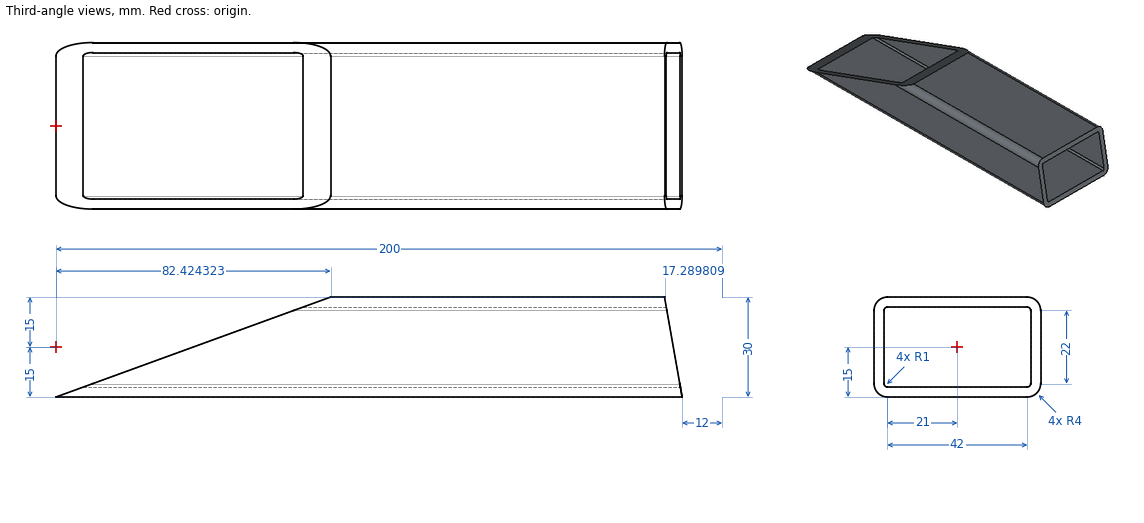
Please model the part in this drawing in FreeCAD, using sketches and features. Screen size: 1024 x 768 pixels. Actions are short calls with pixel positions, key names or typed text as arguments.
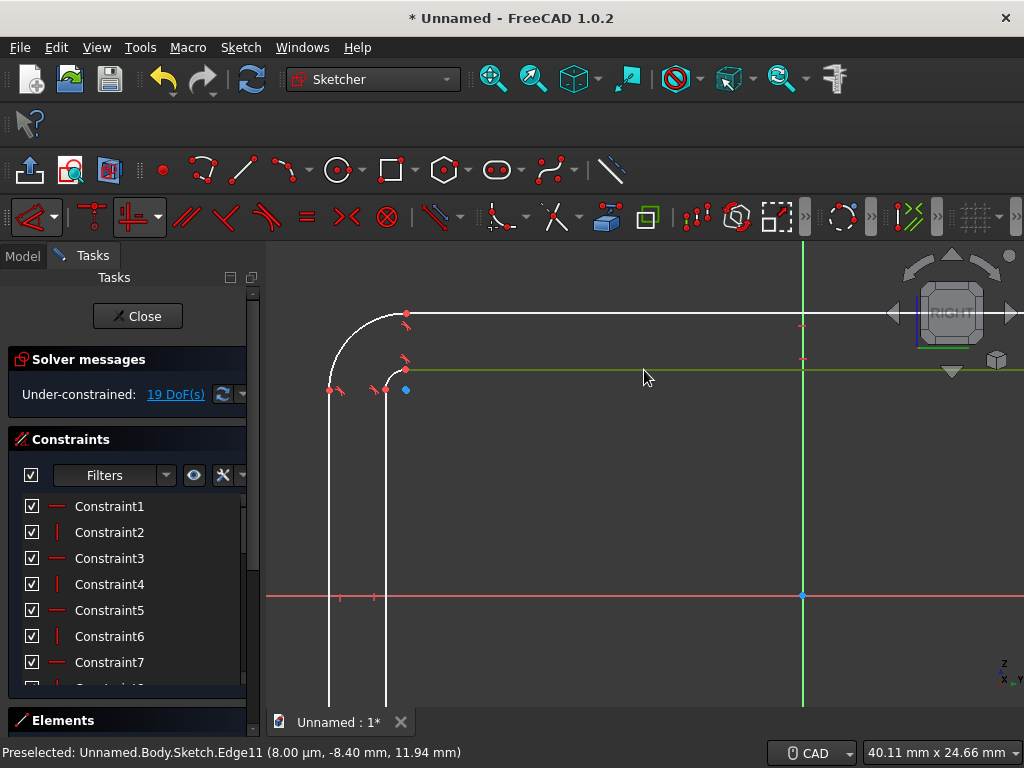
scroll(392, 375, down, 4)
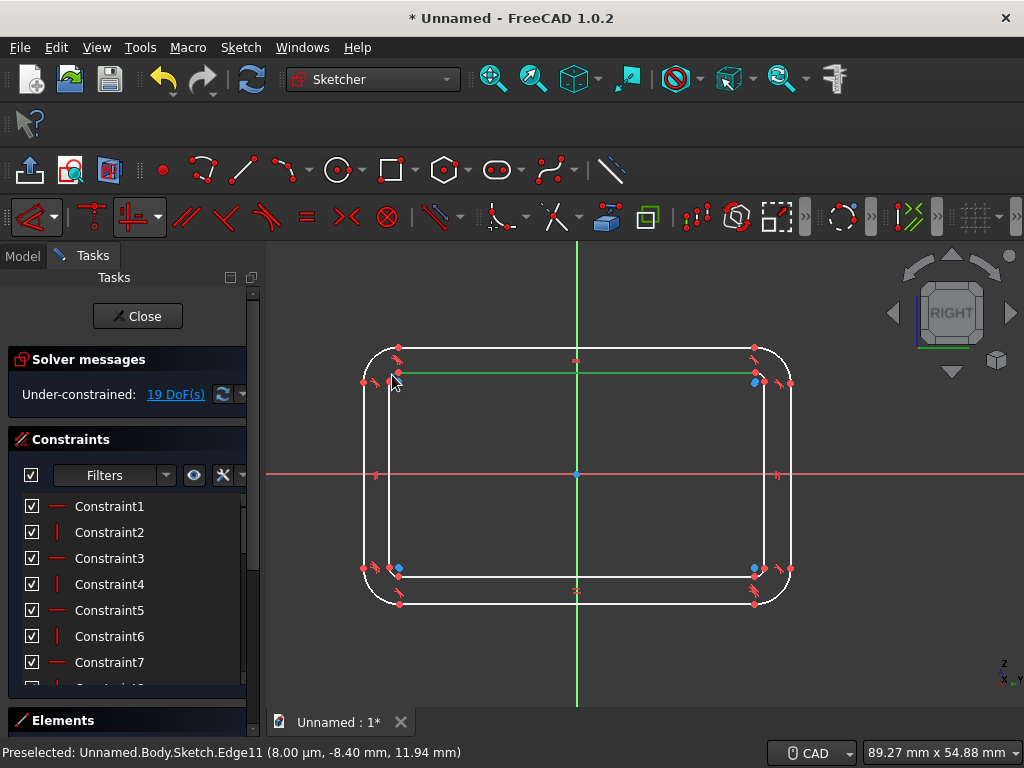
scroll(764, 377, up, 7)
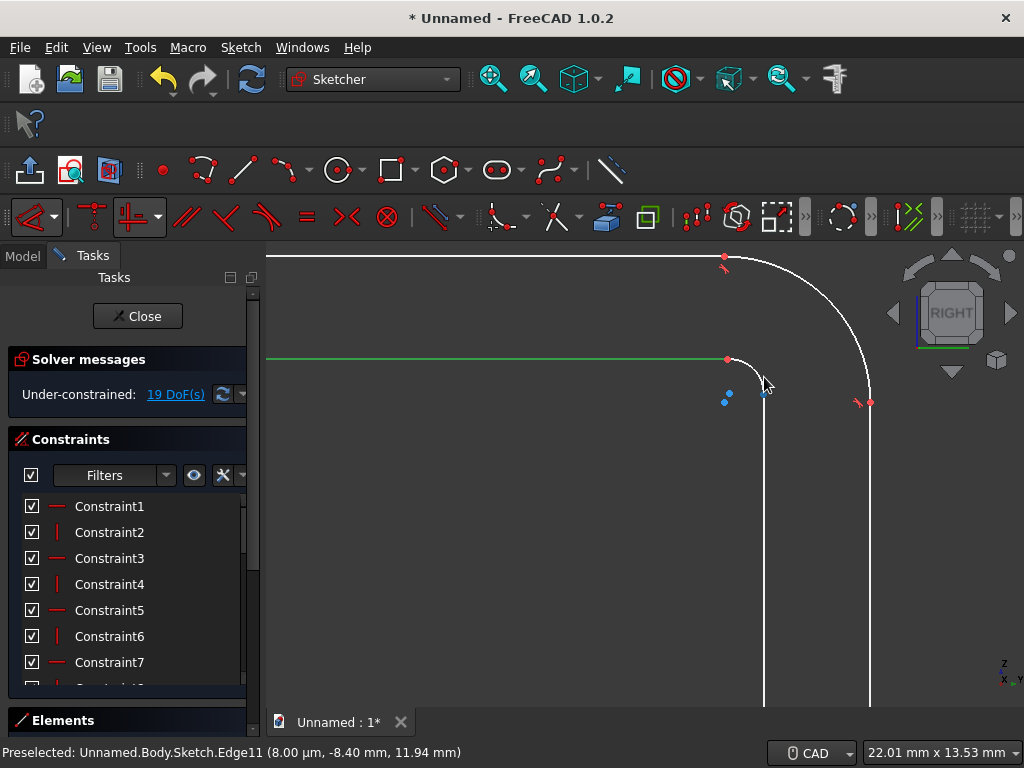
click(760, 378)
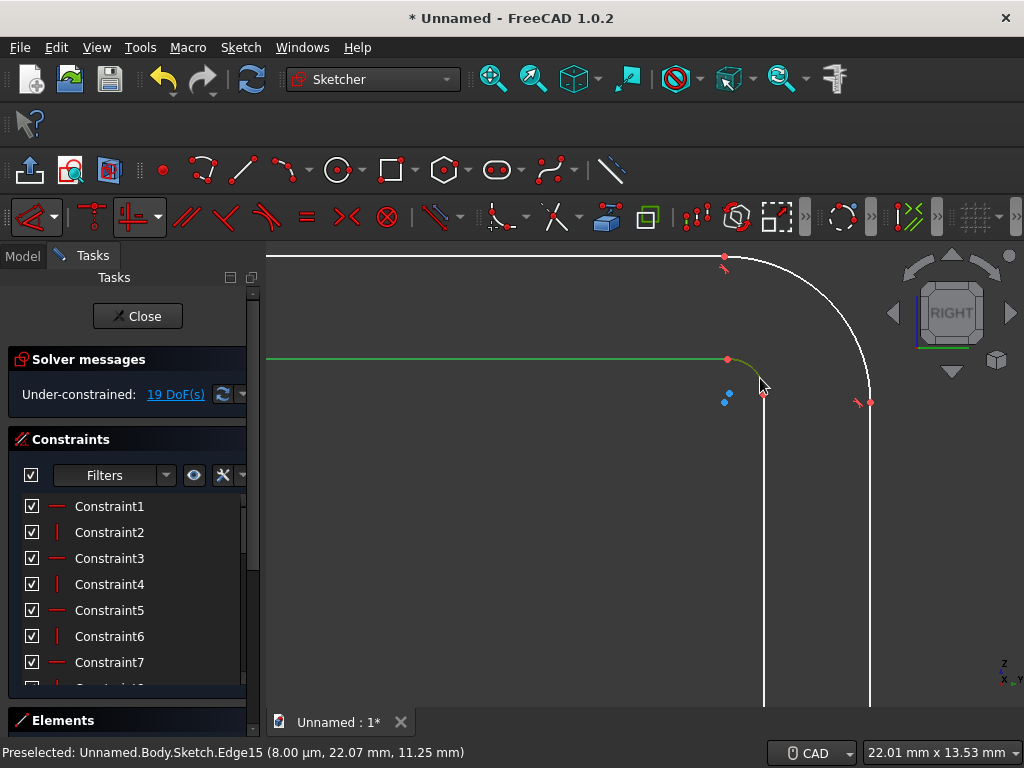
click(268, 218)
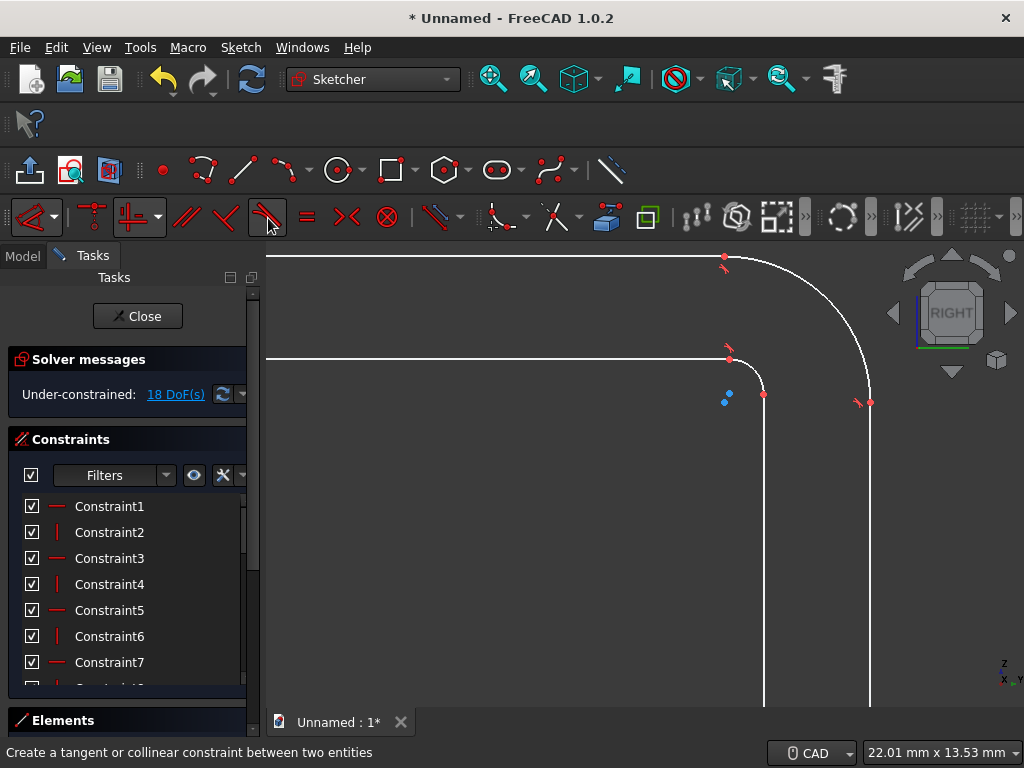
scroll(764, 377, down, 7)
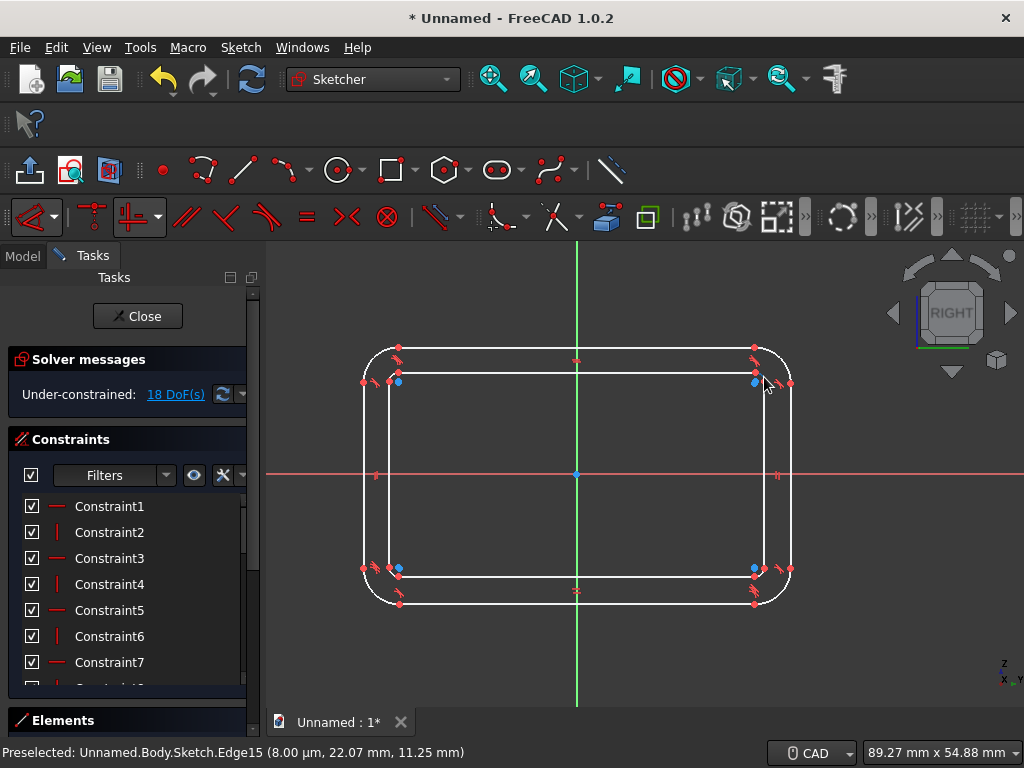
click(764, 437)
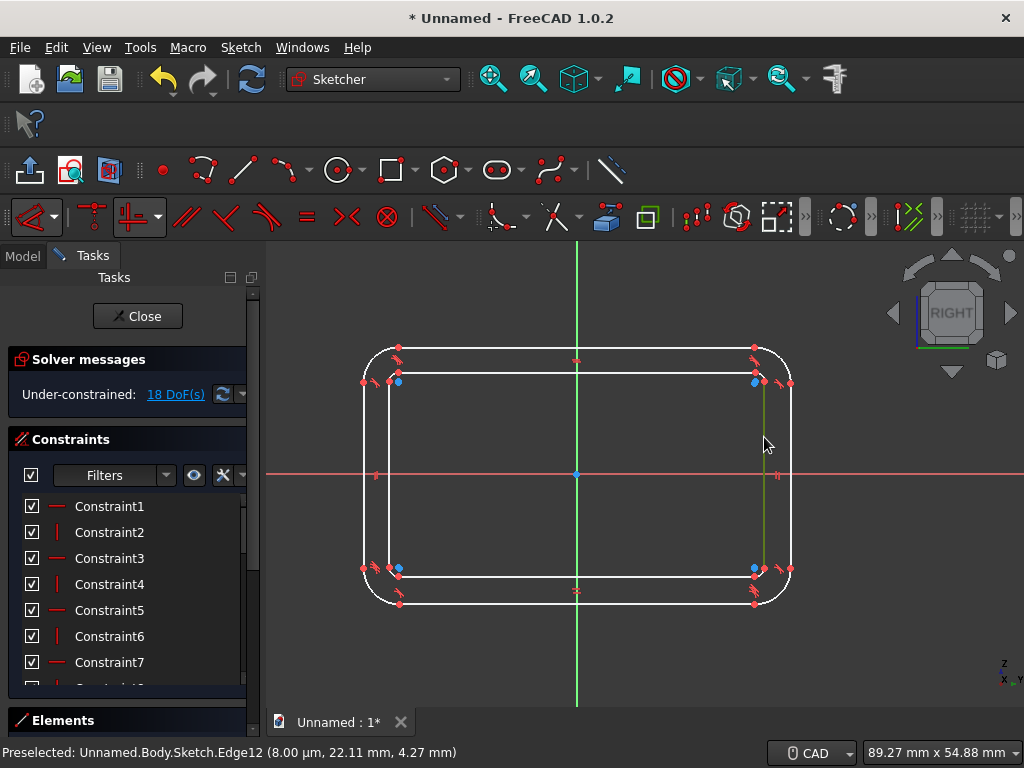
scroll(762, 375, up, 4)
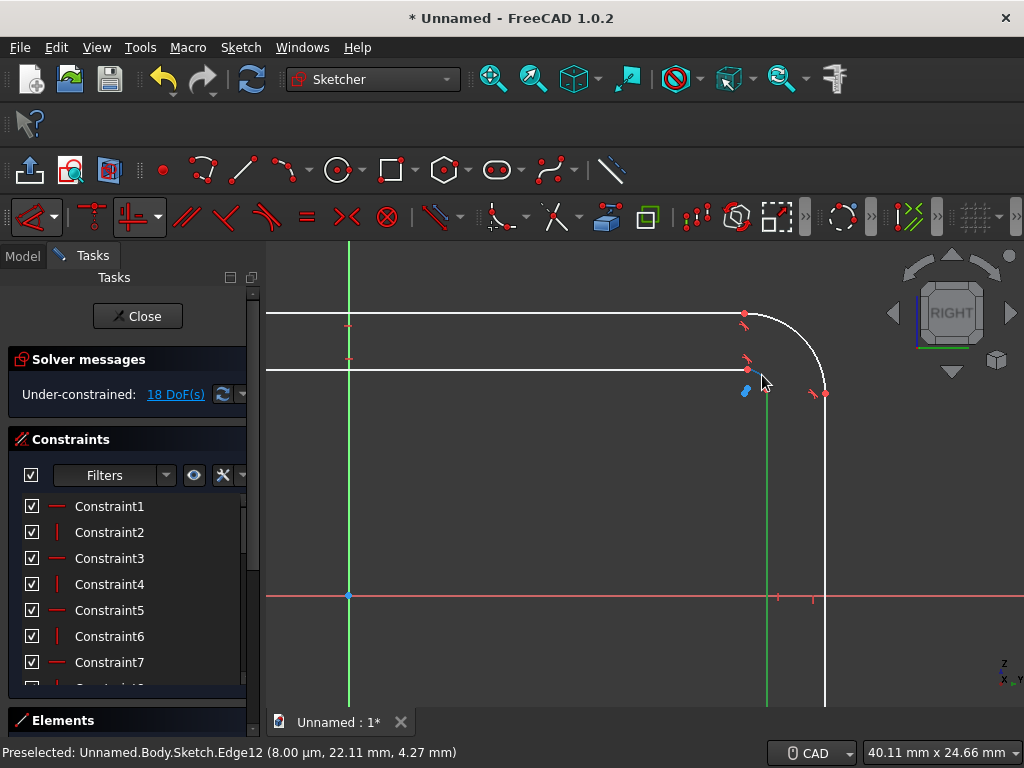
click(761, 376)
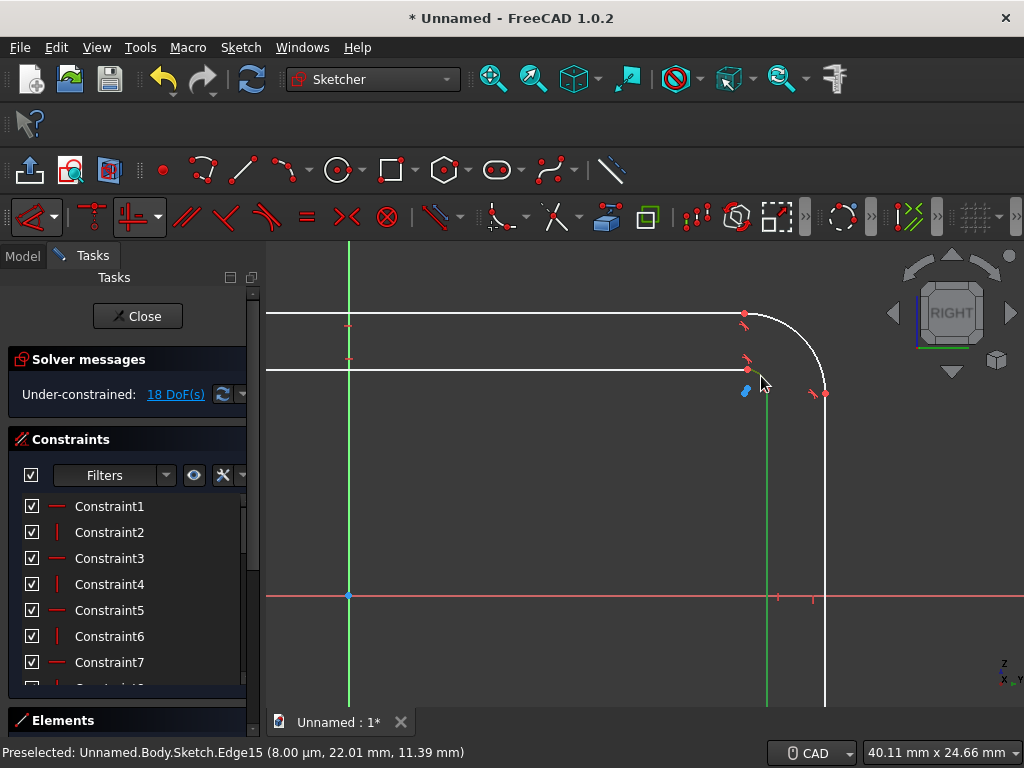
click(268, 218)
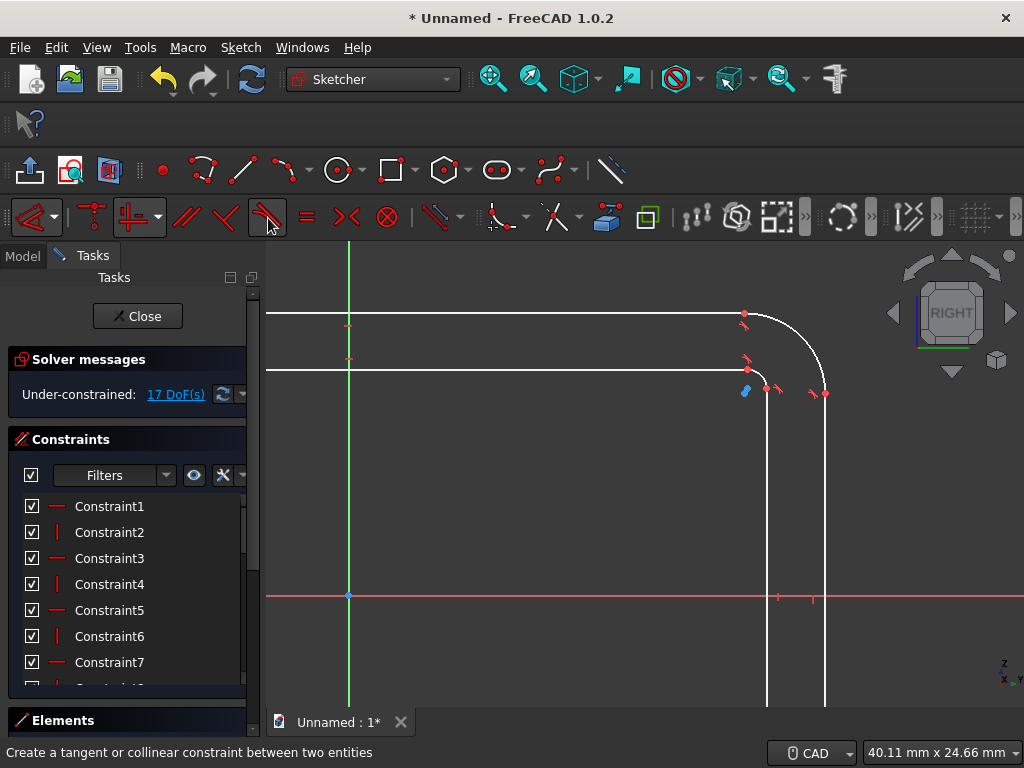
click(767, 513)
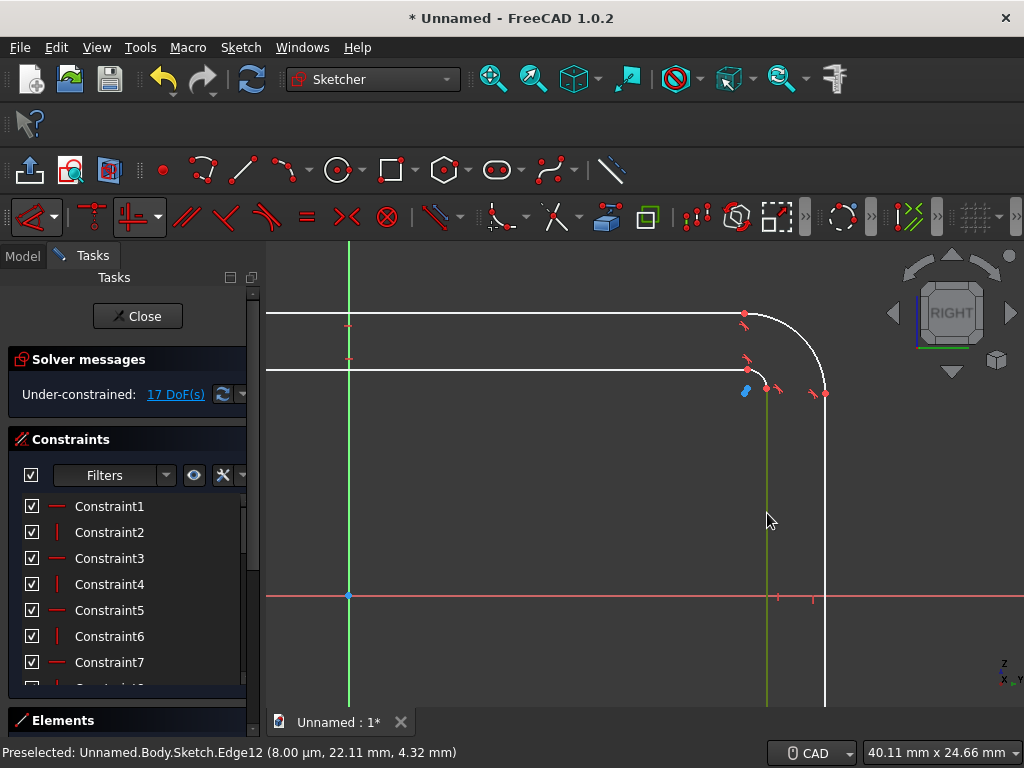
scroll(762, 375, down, 4)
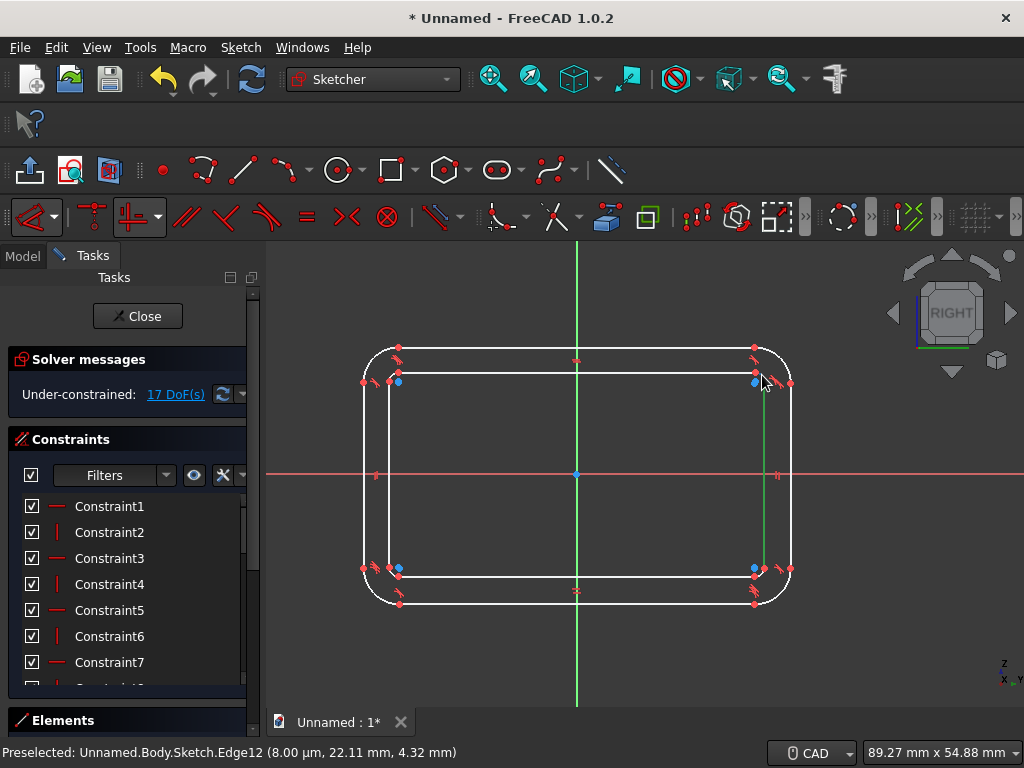
scroll(759, 576, up, 6)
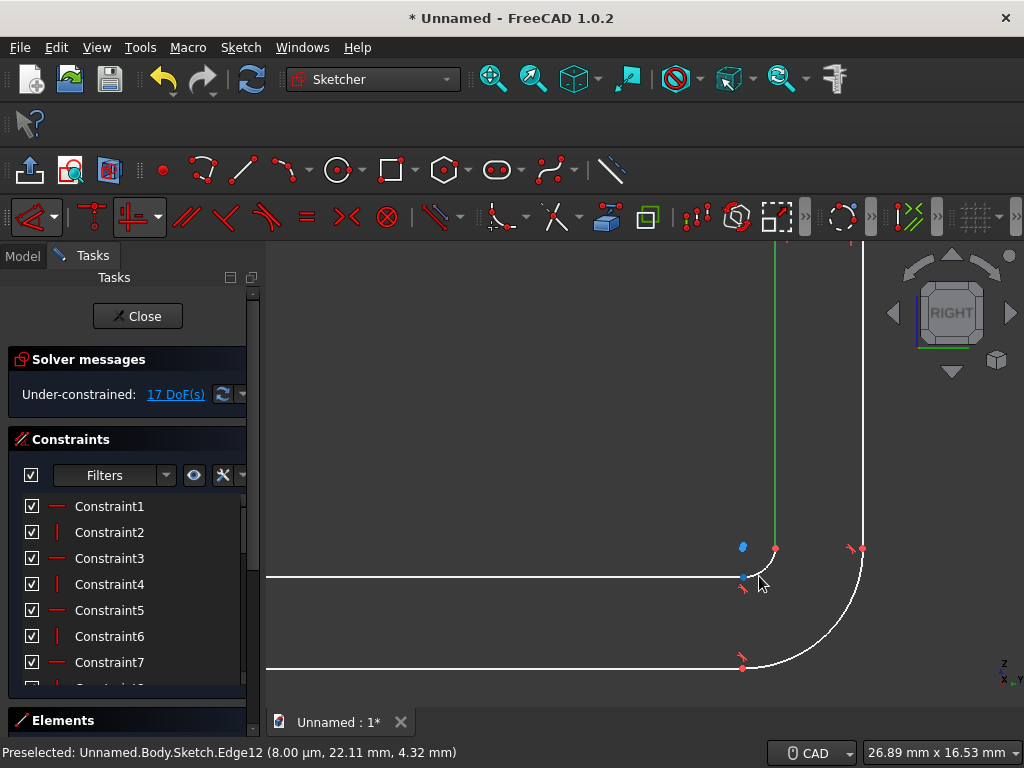
click(757, 574)